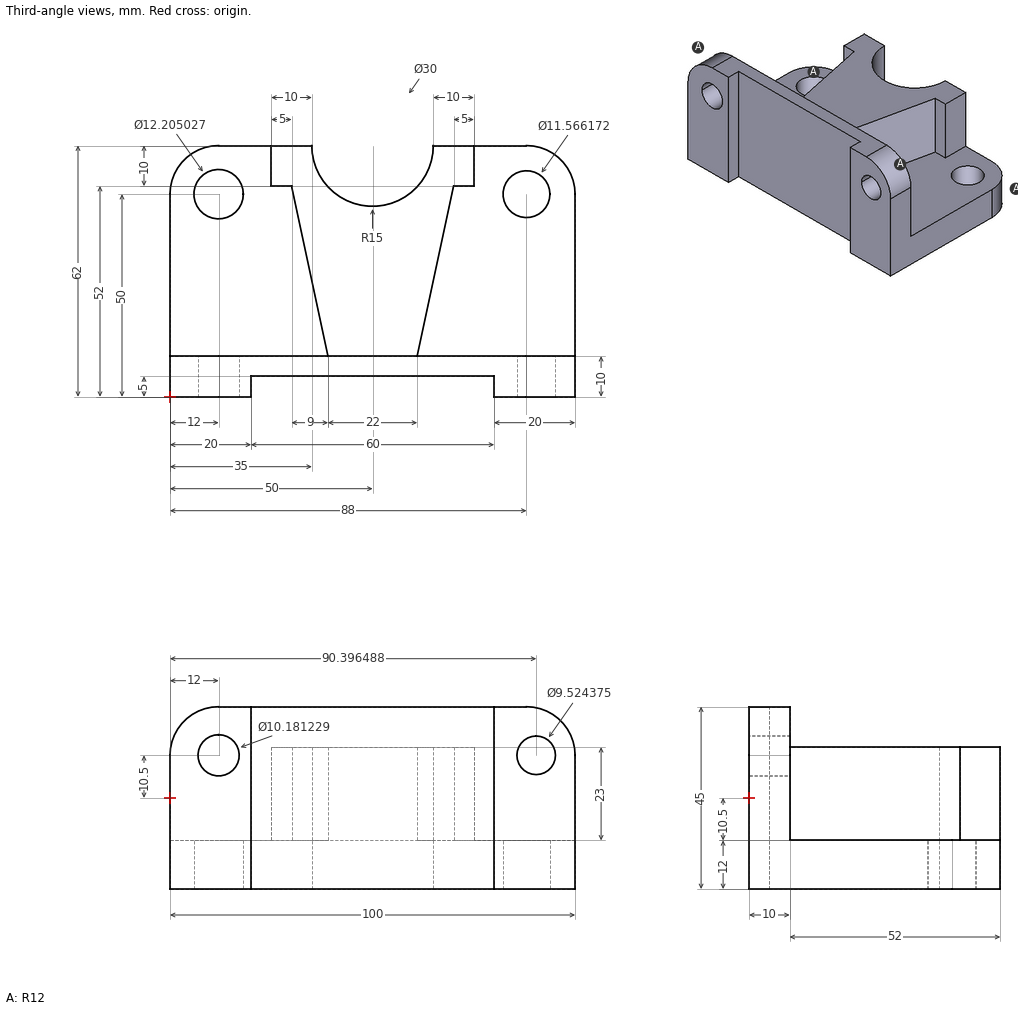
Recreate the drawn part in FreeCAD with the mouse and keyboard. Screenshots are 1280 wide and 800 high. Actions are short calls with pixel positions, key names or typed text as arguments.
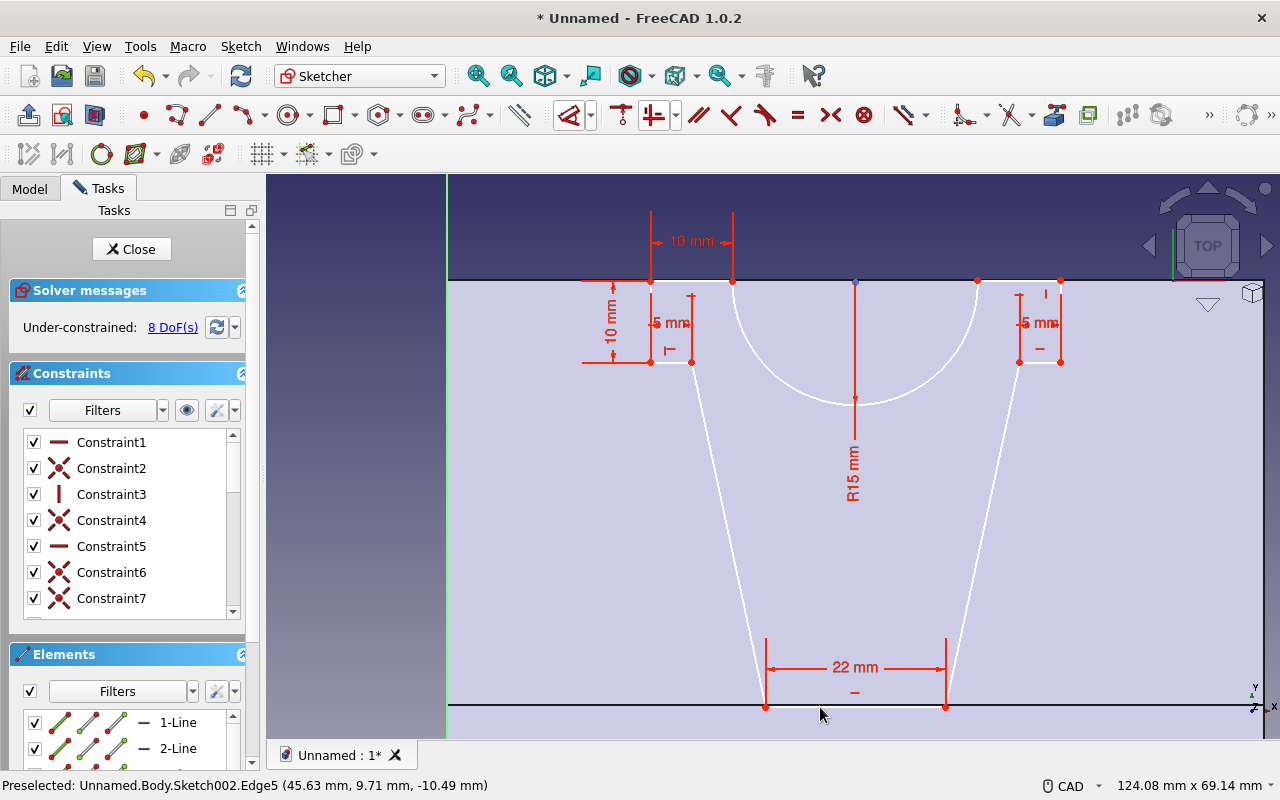
click(1061, 338)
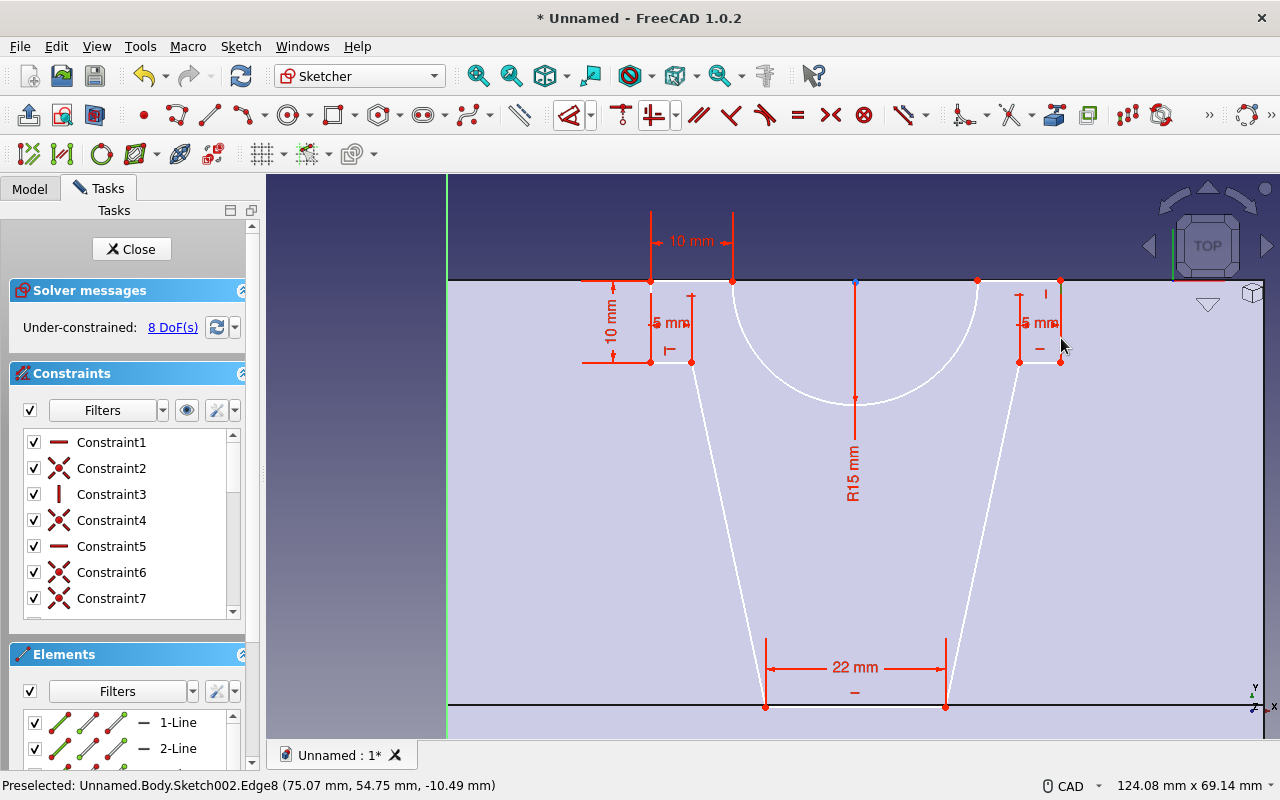
key(i)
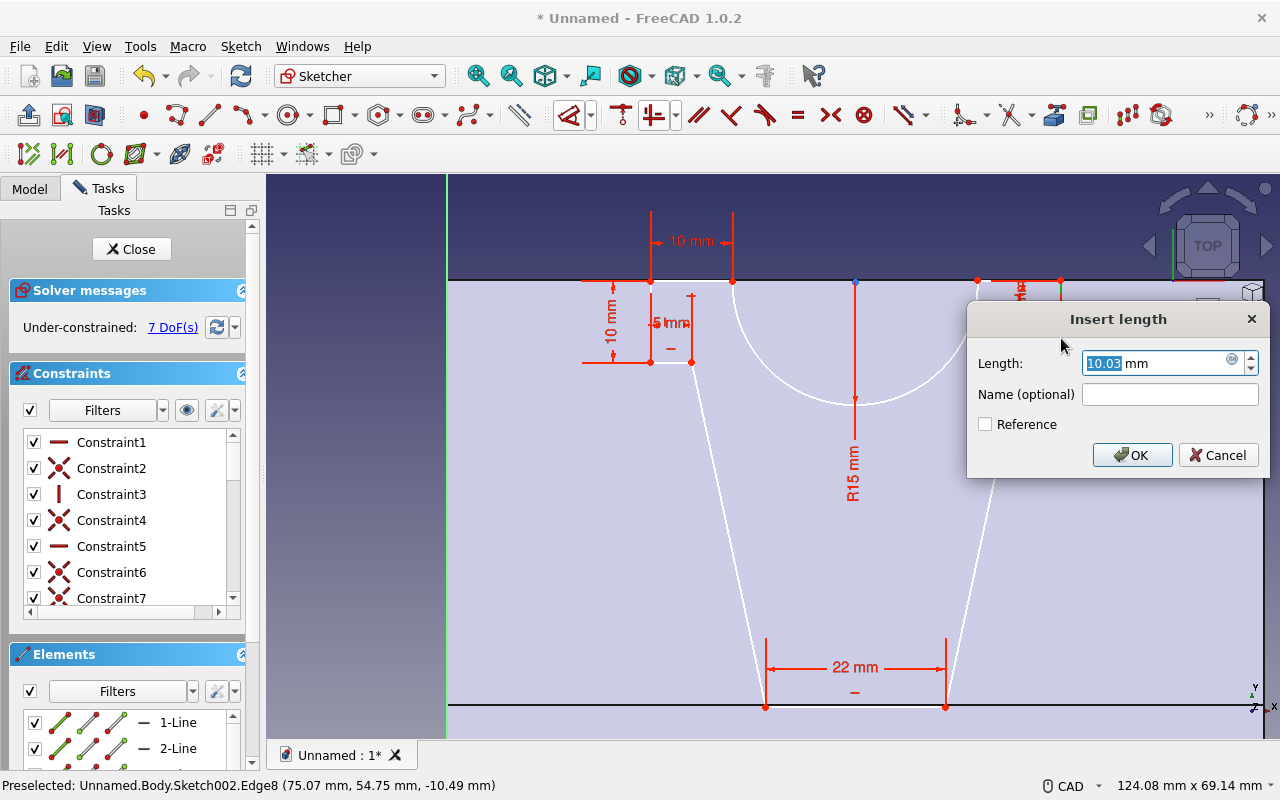
text(10)
key(Return)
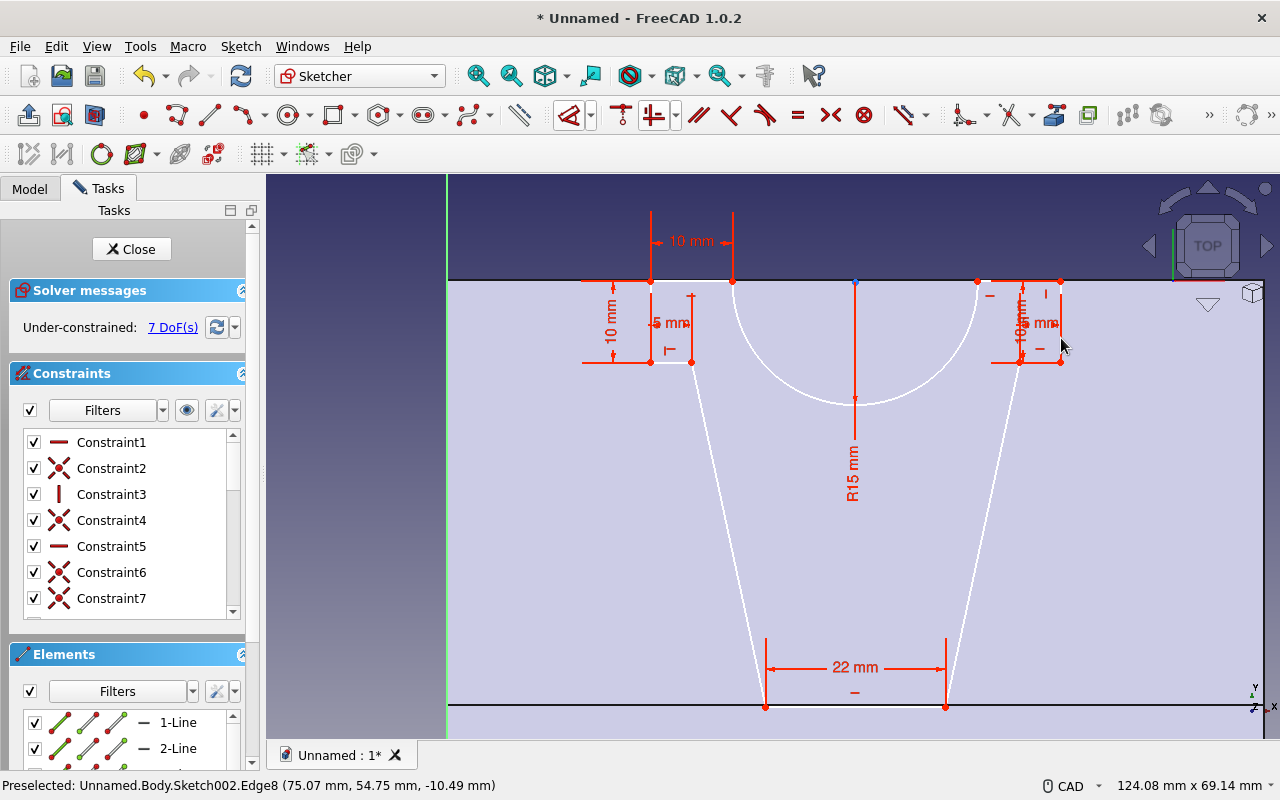
click(1036, 281)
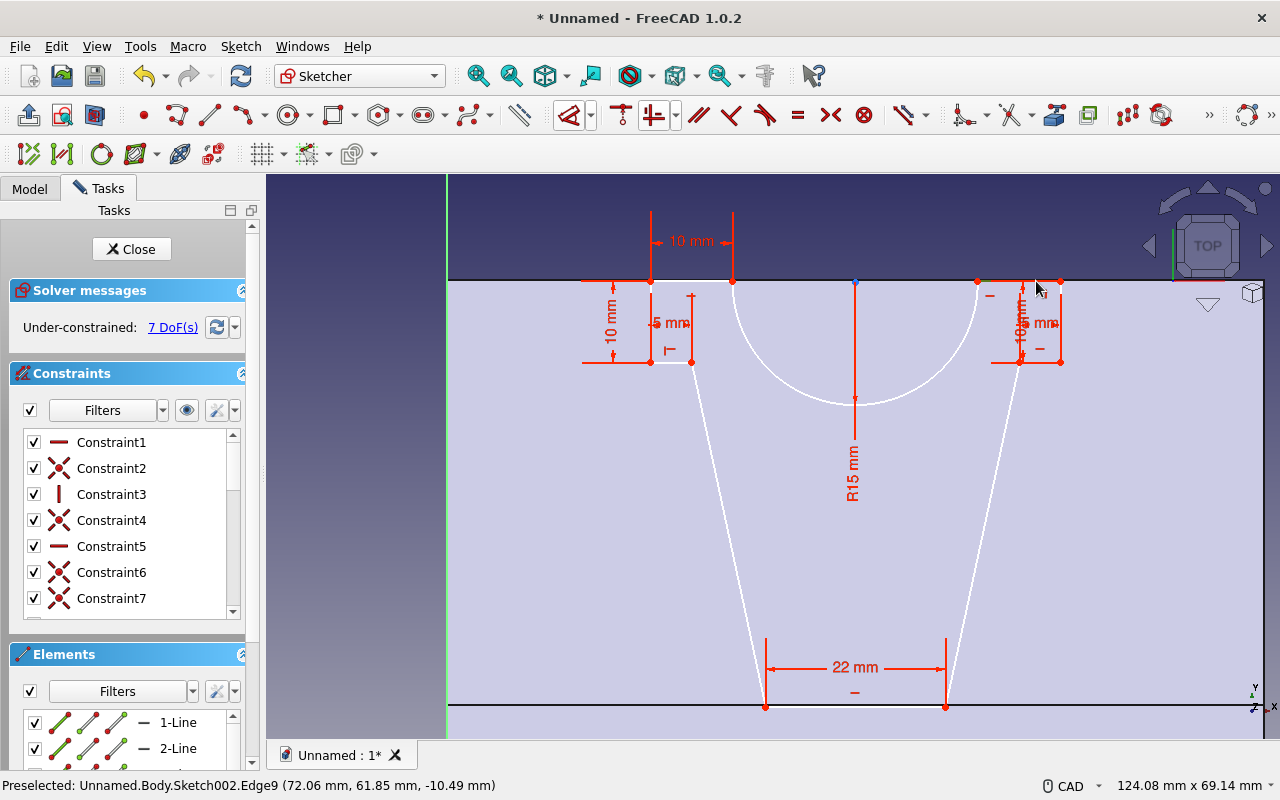
key(l)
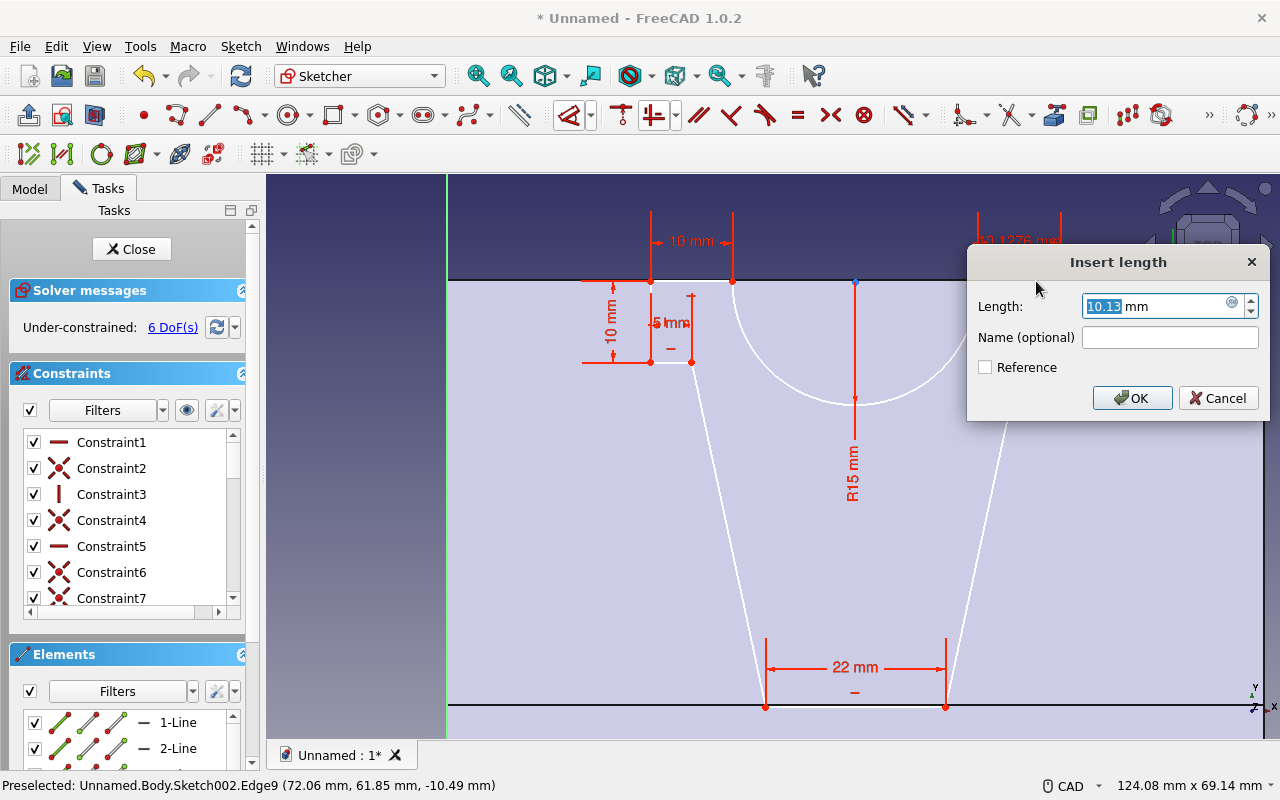
text(10)
key(Return)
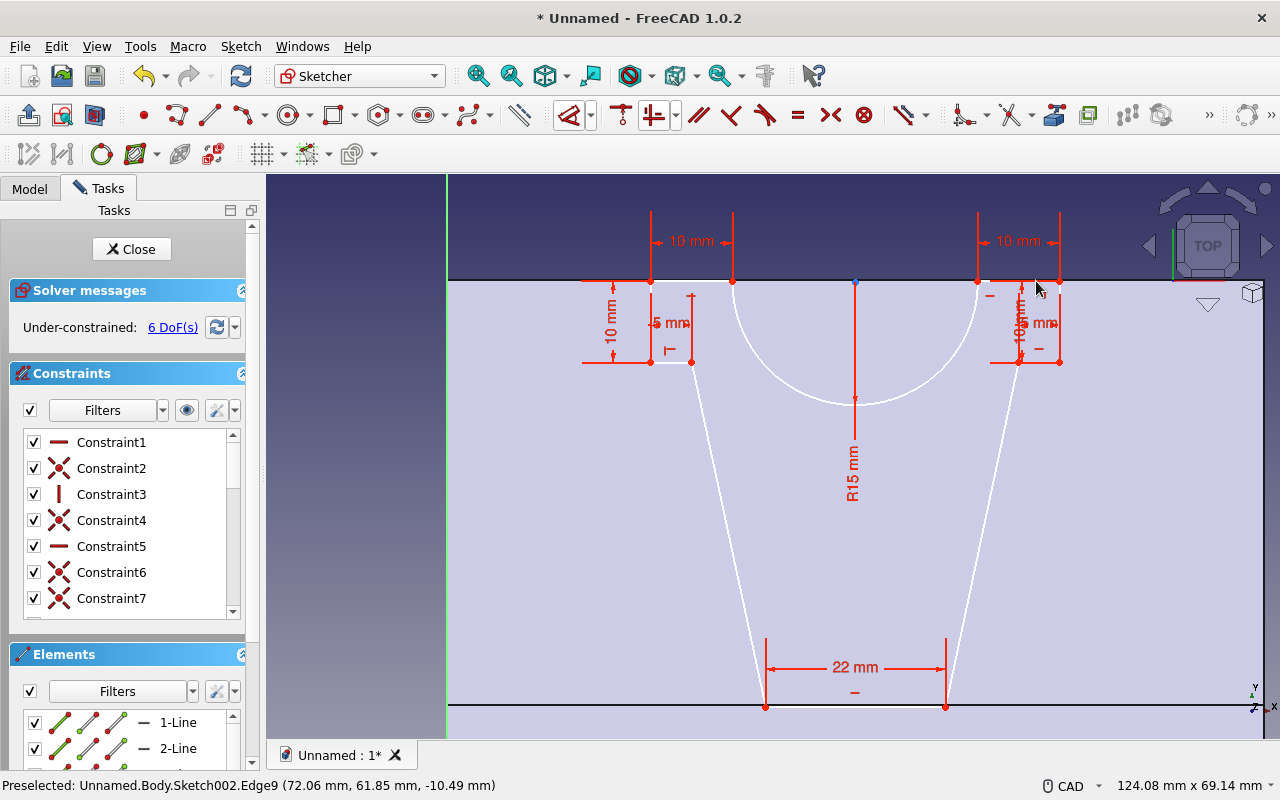
click(714, 466)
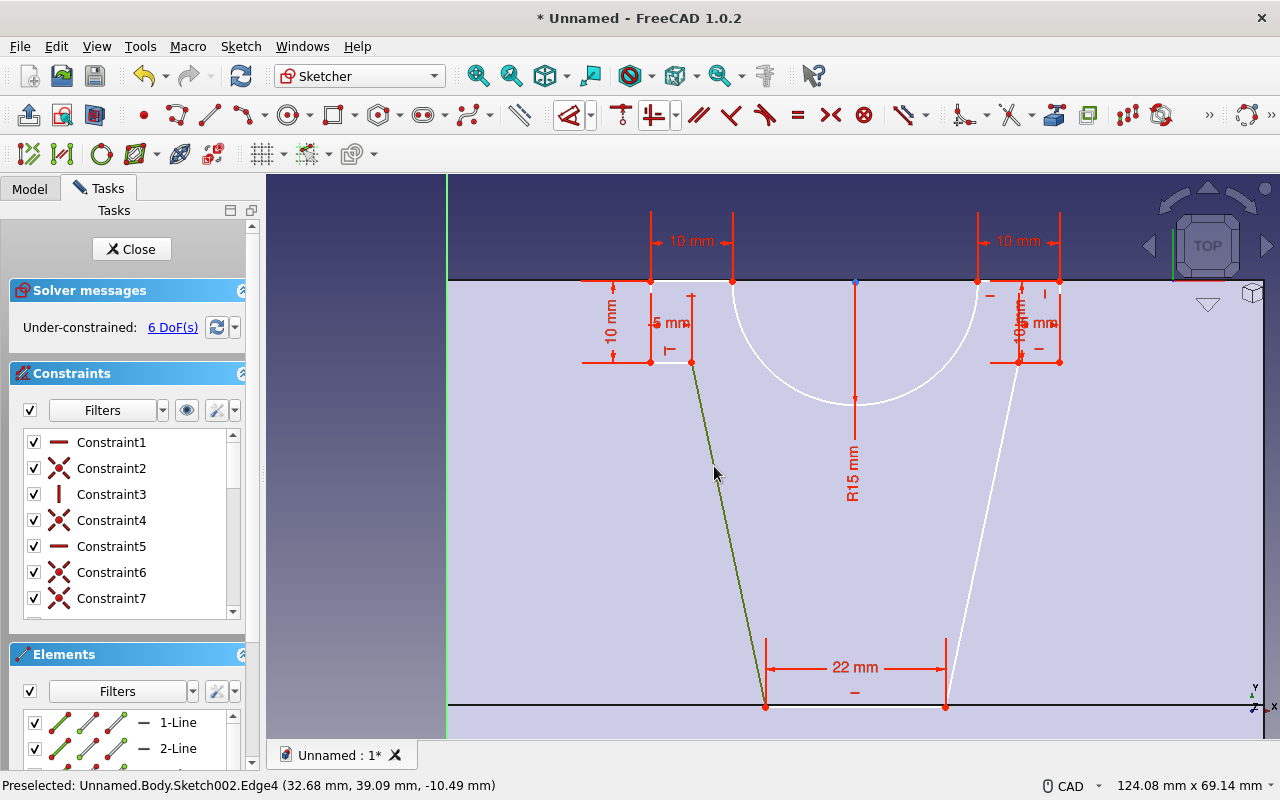
key(l)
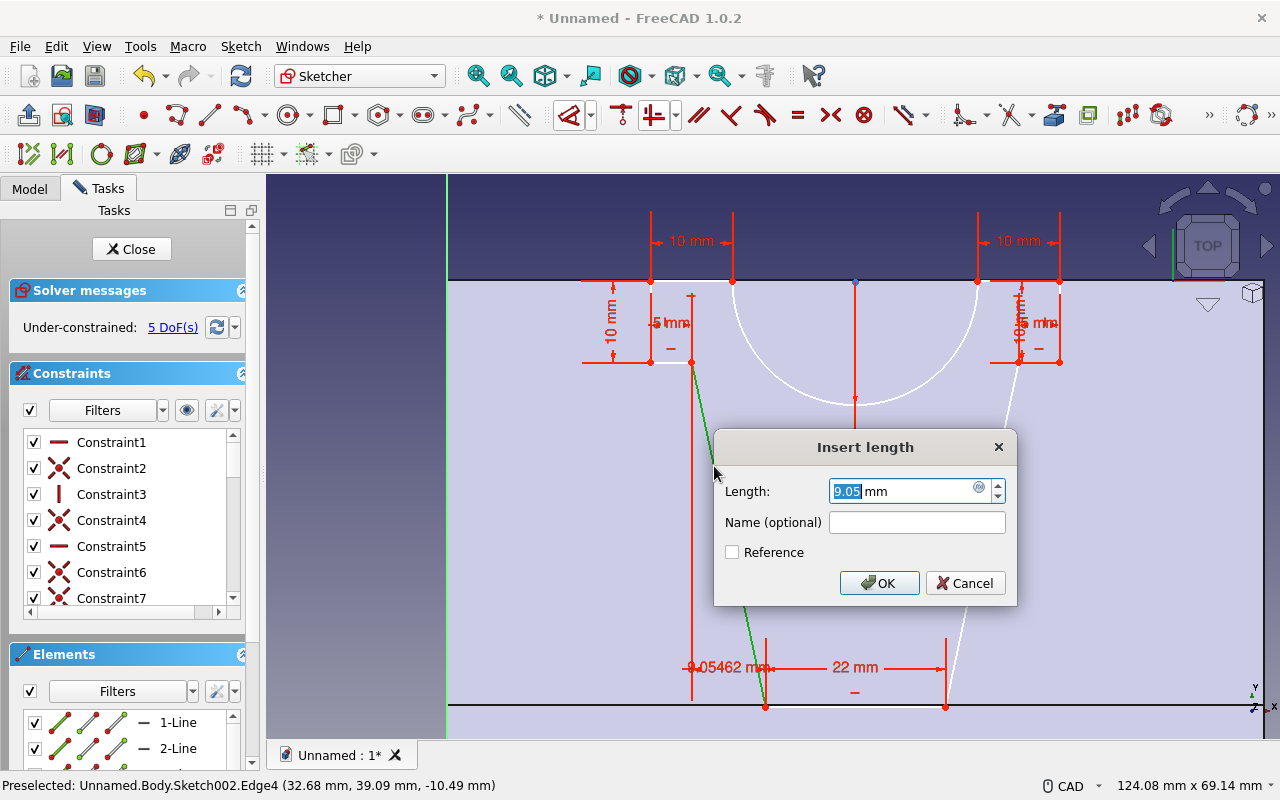
text(9)
key(Return)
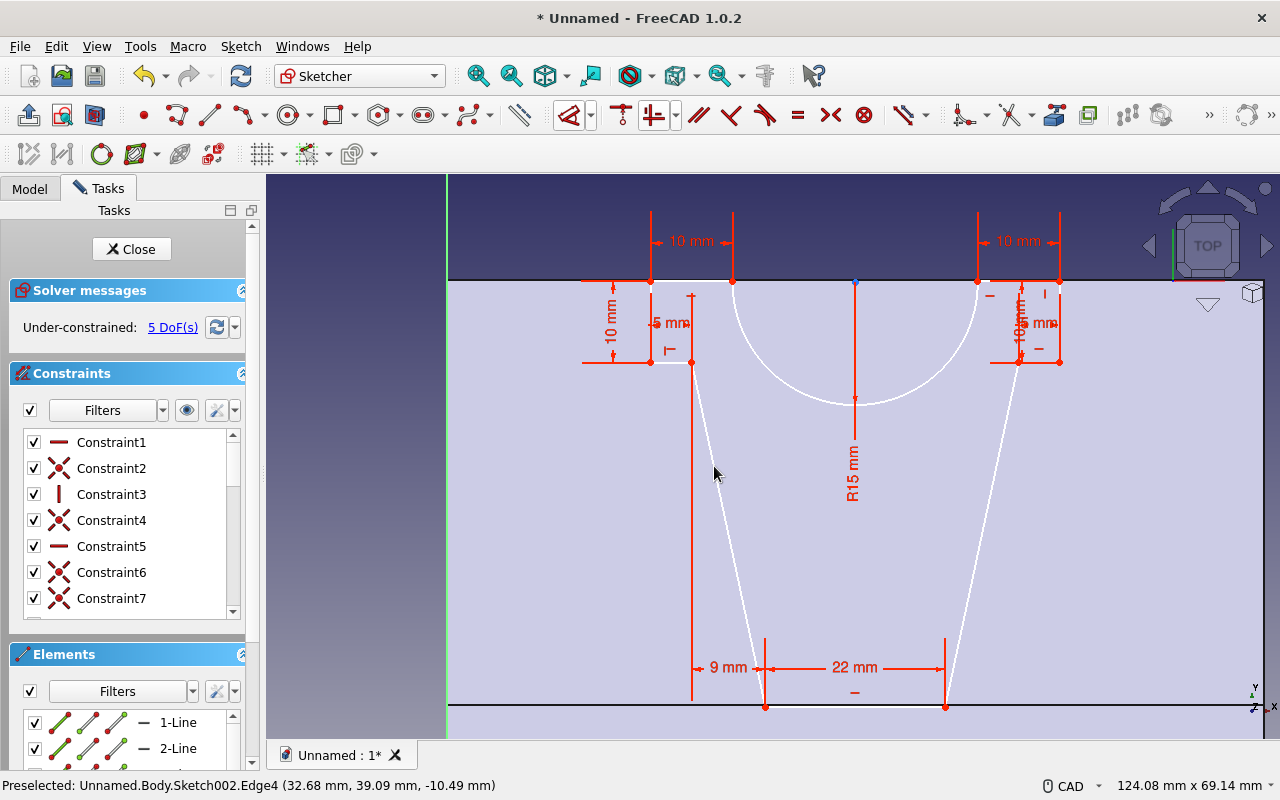
click(733, 281)